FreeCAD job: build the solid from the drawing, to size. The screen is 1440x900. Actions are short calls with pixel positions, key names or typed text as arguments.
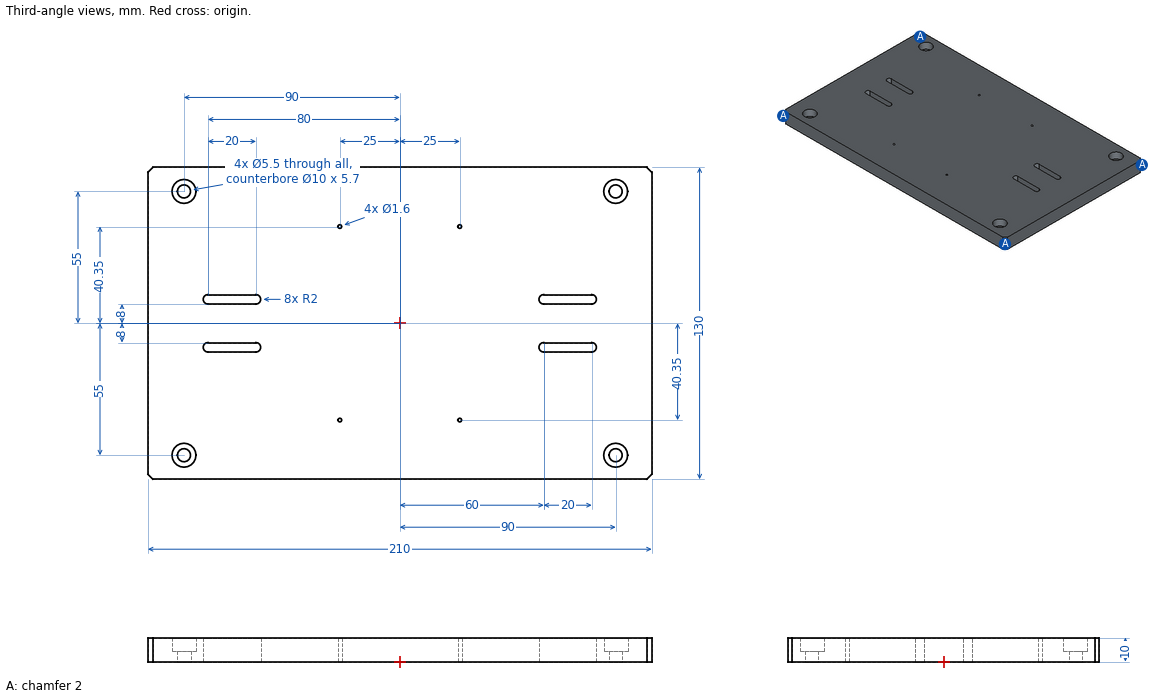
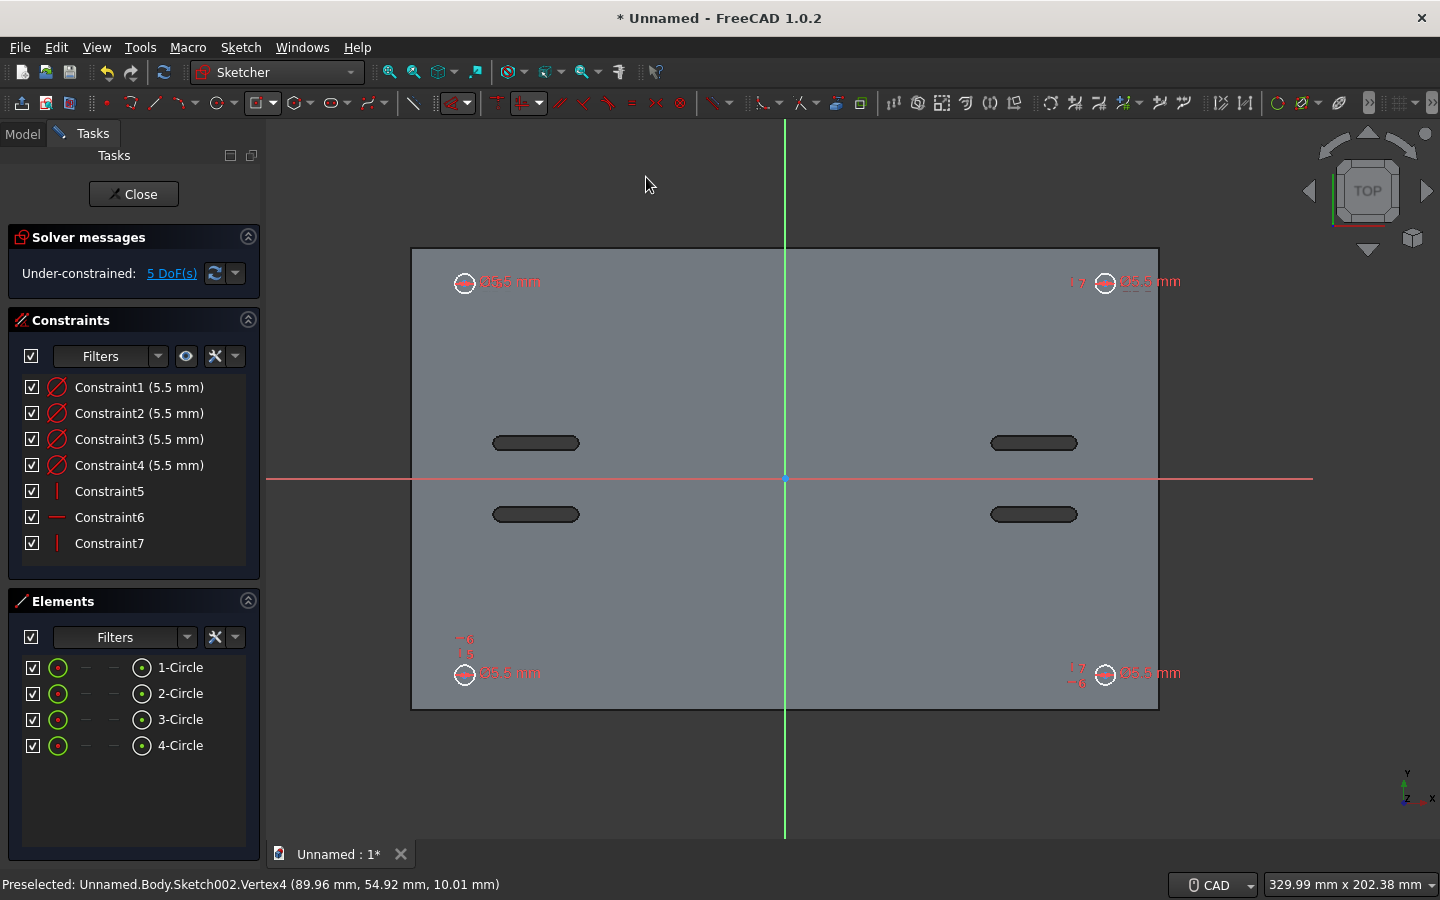
click(465, 284)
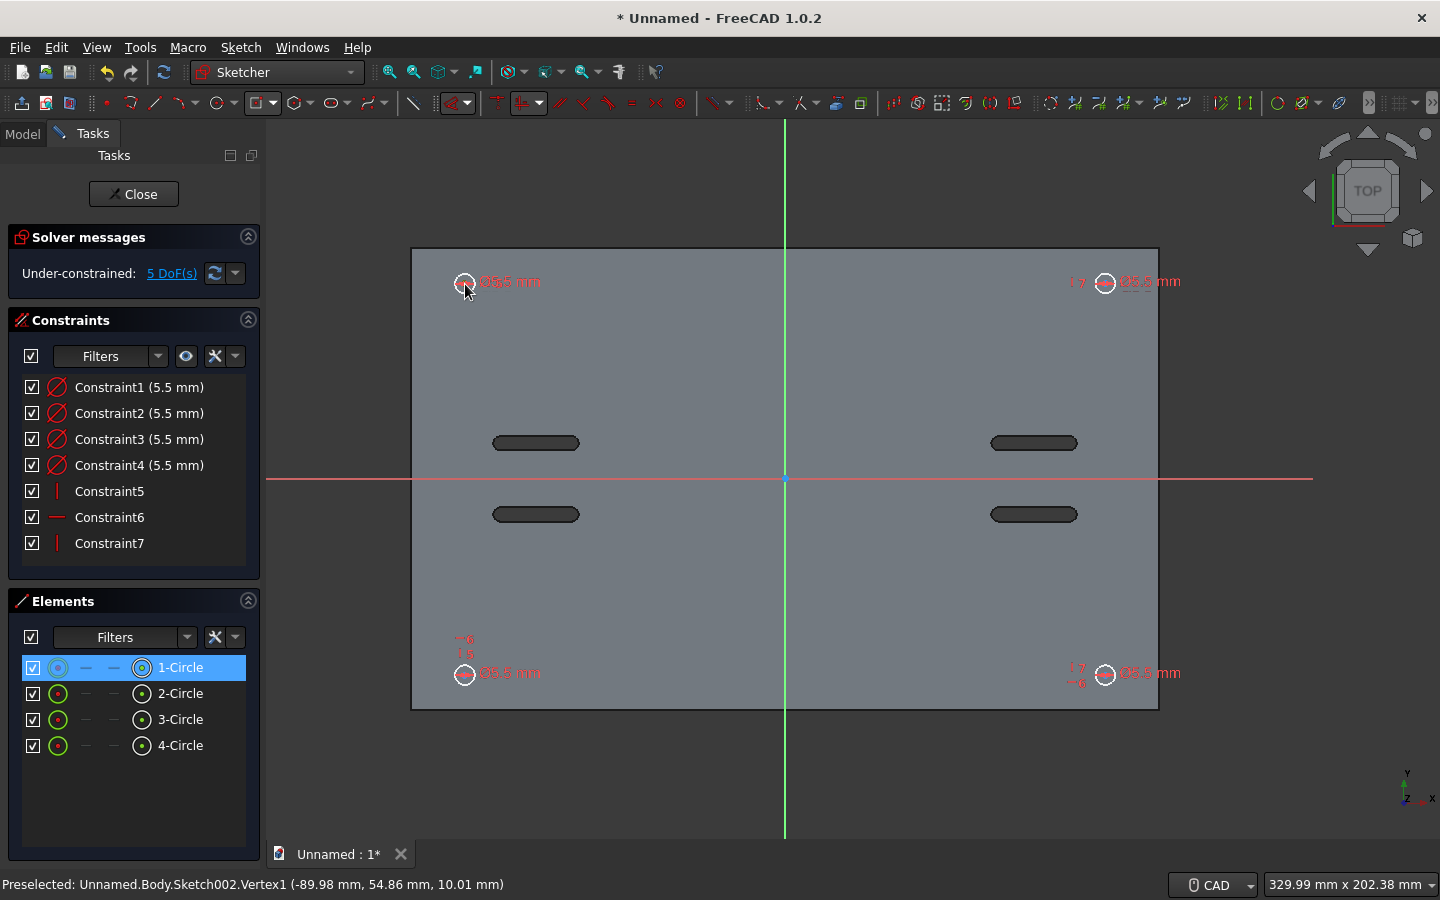
click(1105, 284)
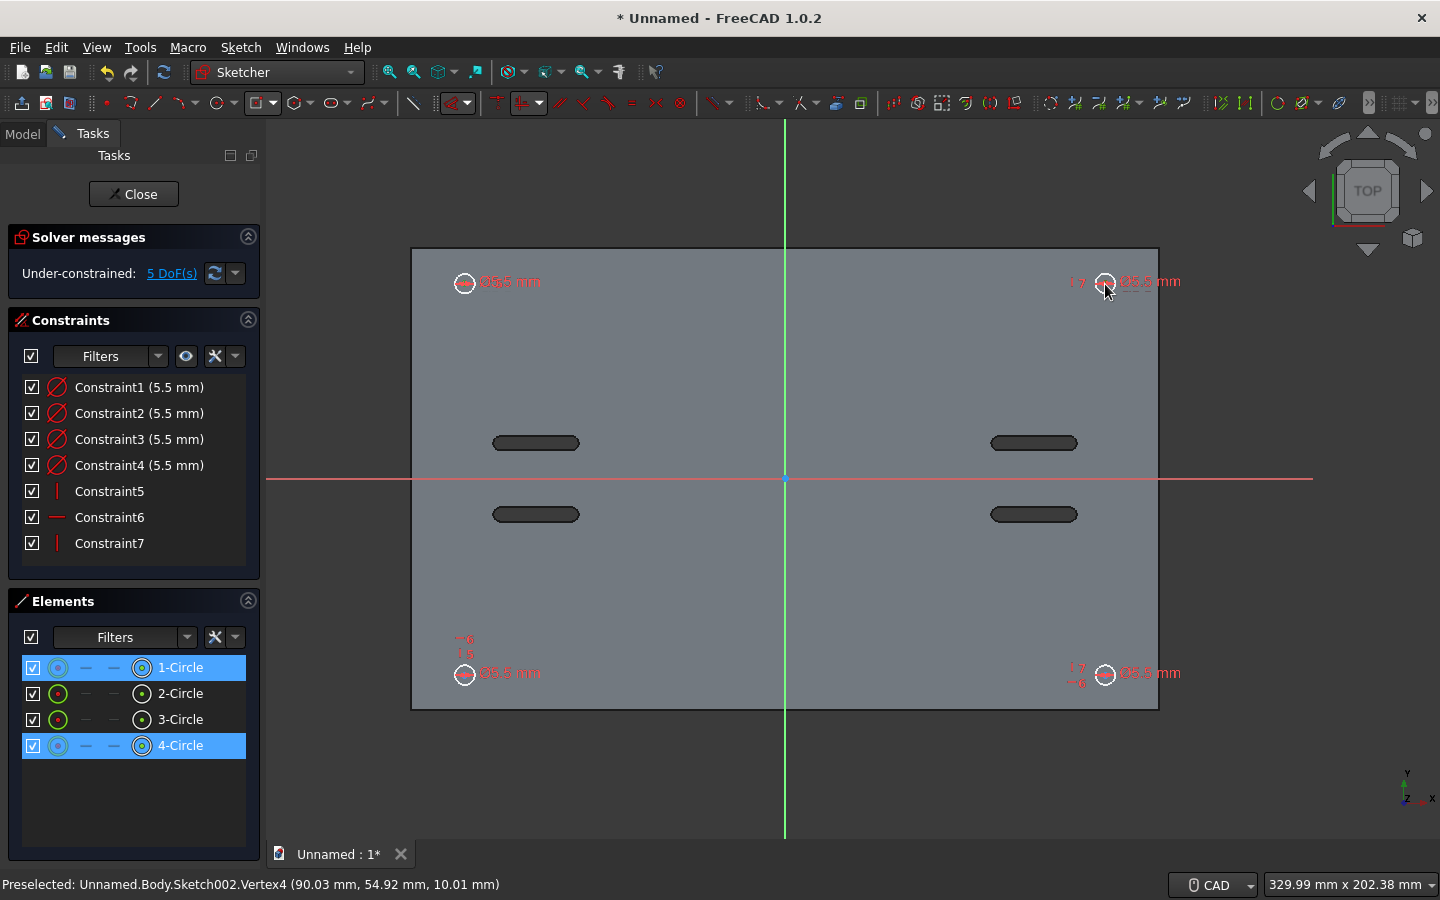
click(542, 104)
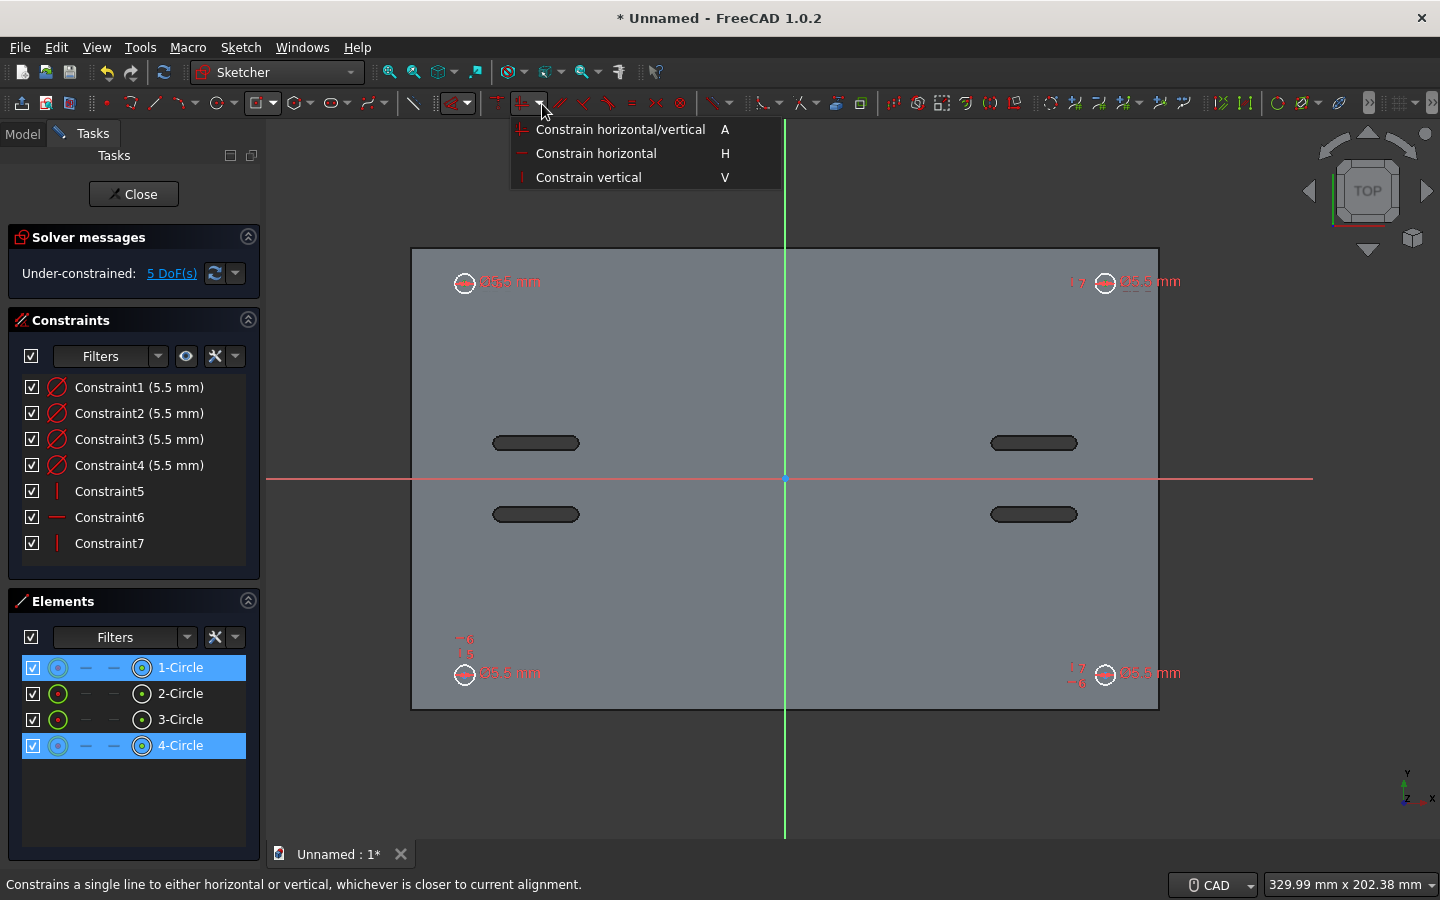
click(646, 153)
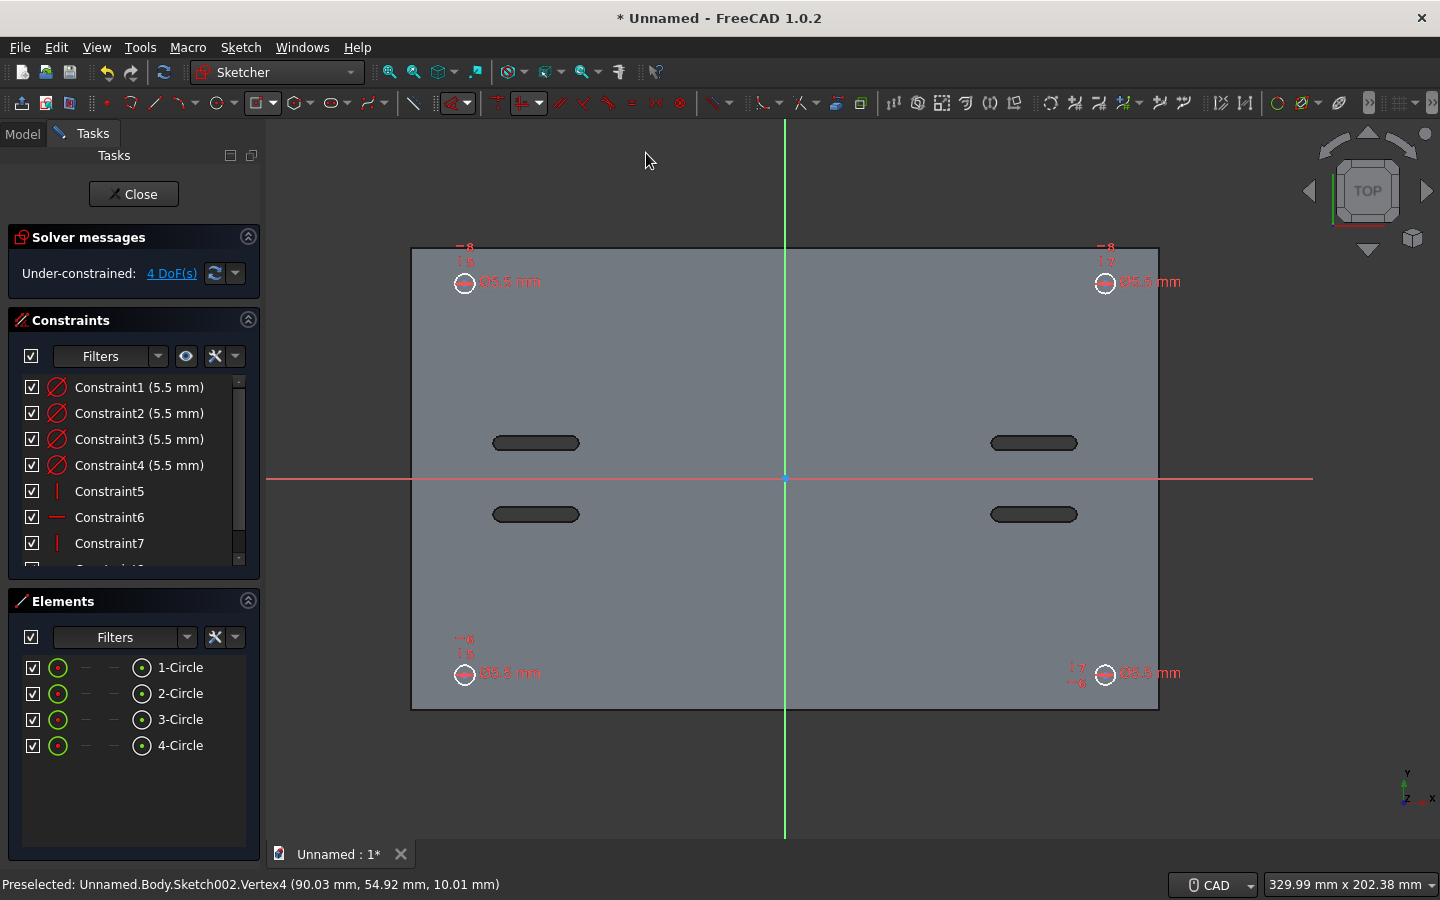
click(465, 284)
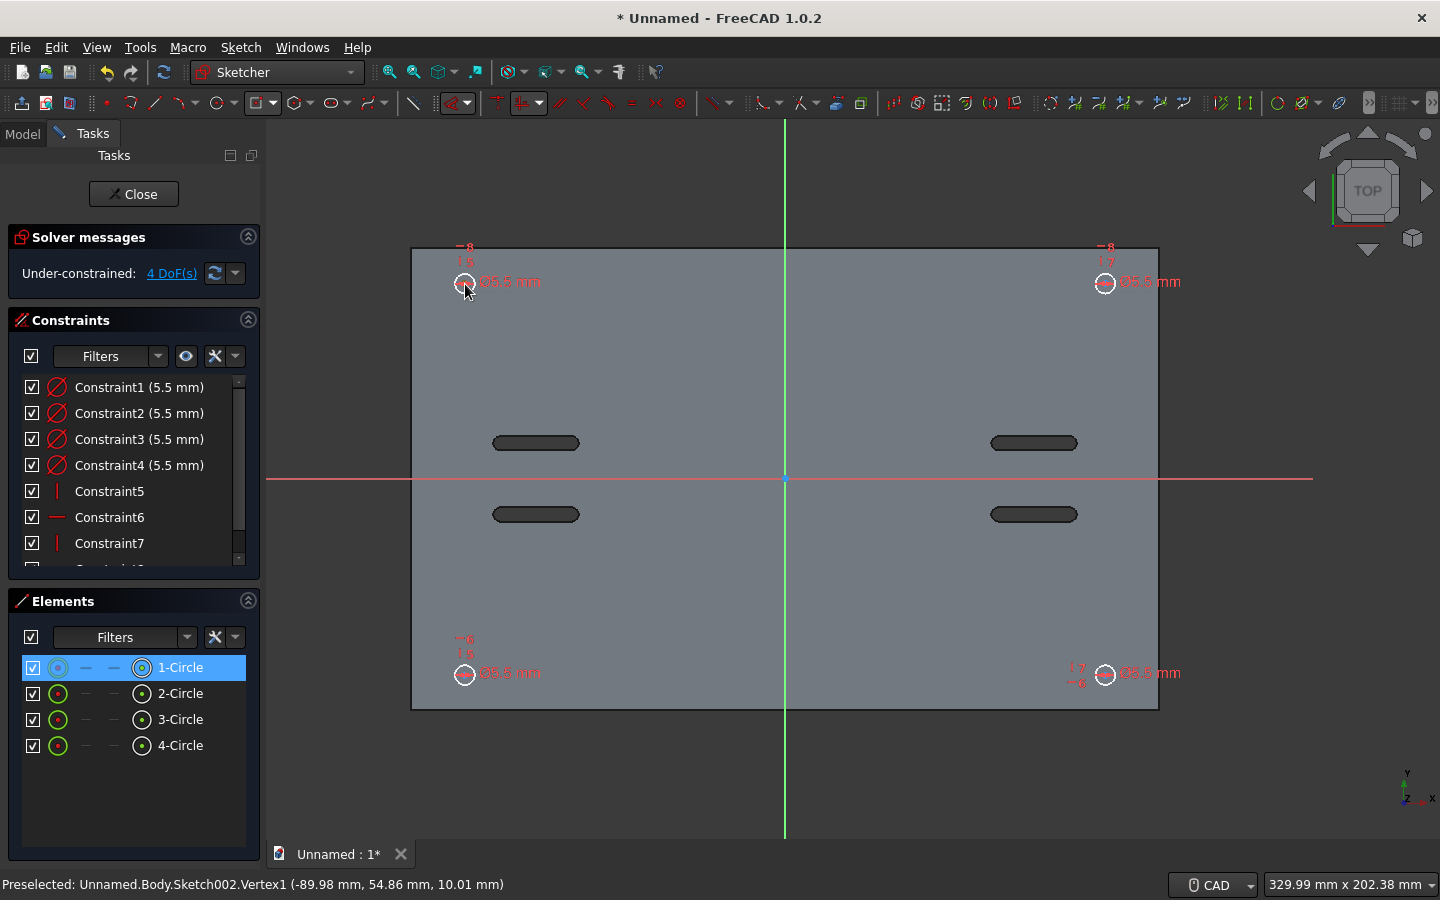
click(470, 104)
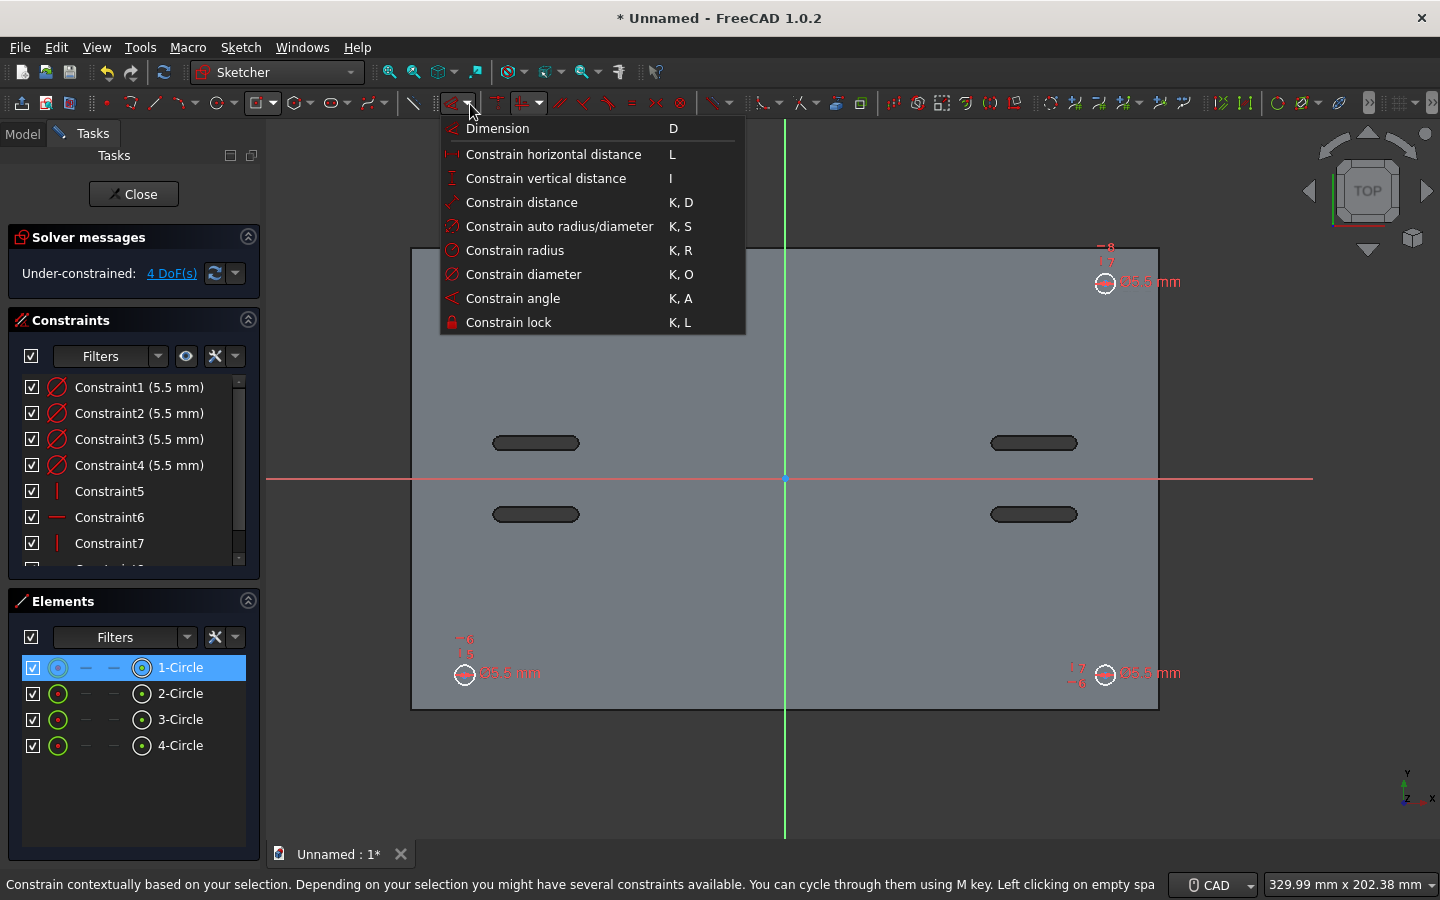
click(593, 154)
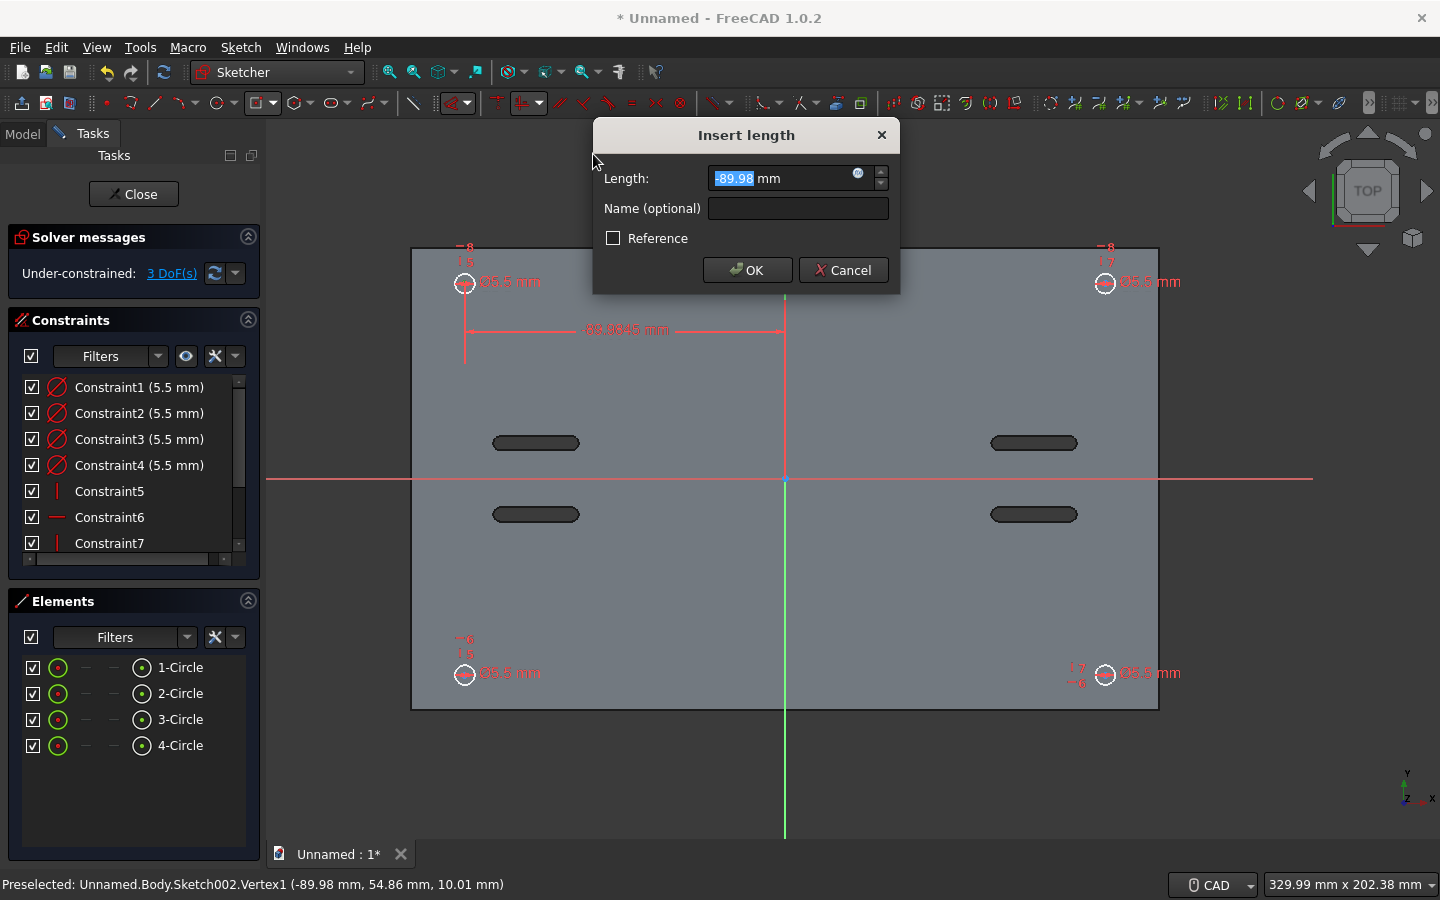
text(-90)
key(Return)